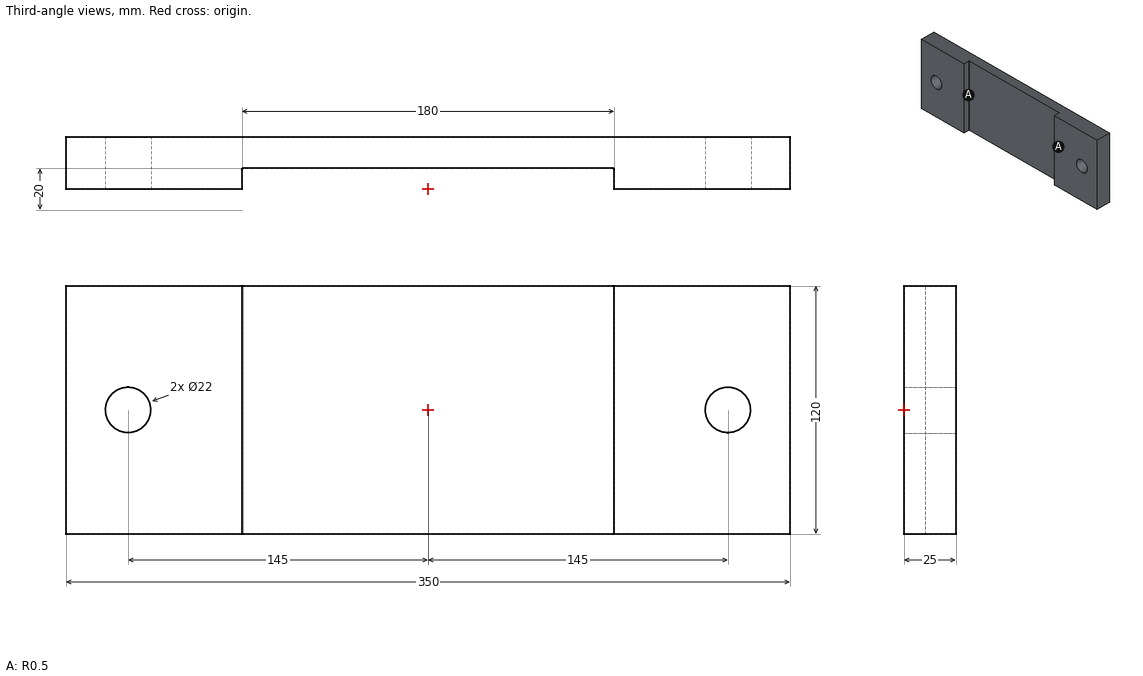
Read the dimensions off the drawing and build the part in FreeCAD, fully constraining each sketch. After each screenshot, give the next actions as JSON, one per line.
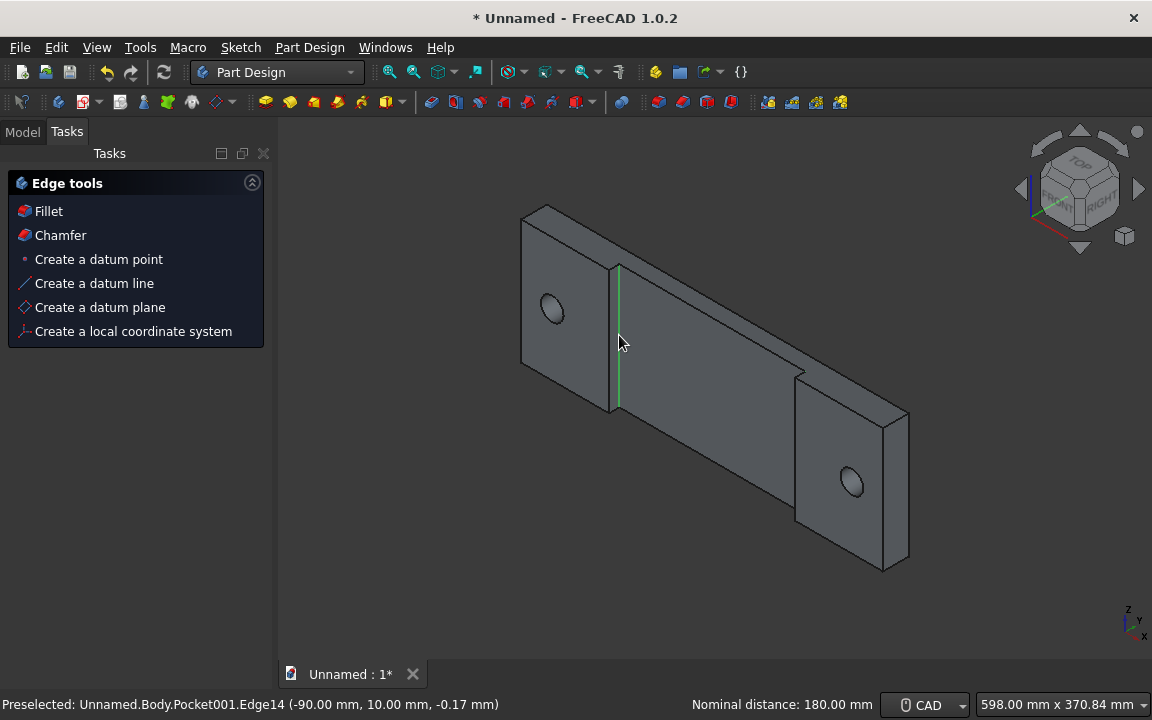
{"action": "left_click", "coordinate": [660, 102]}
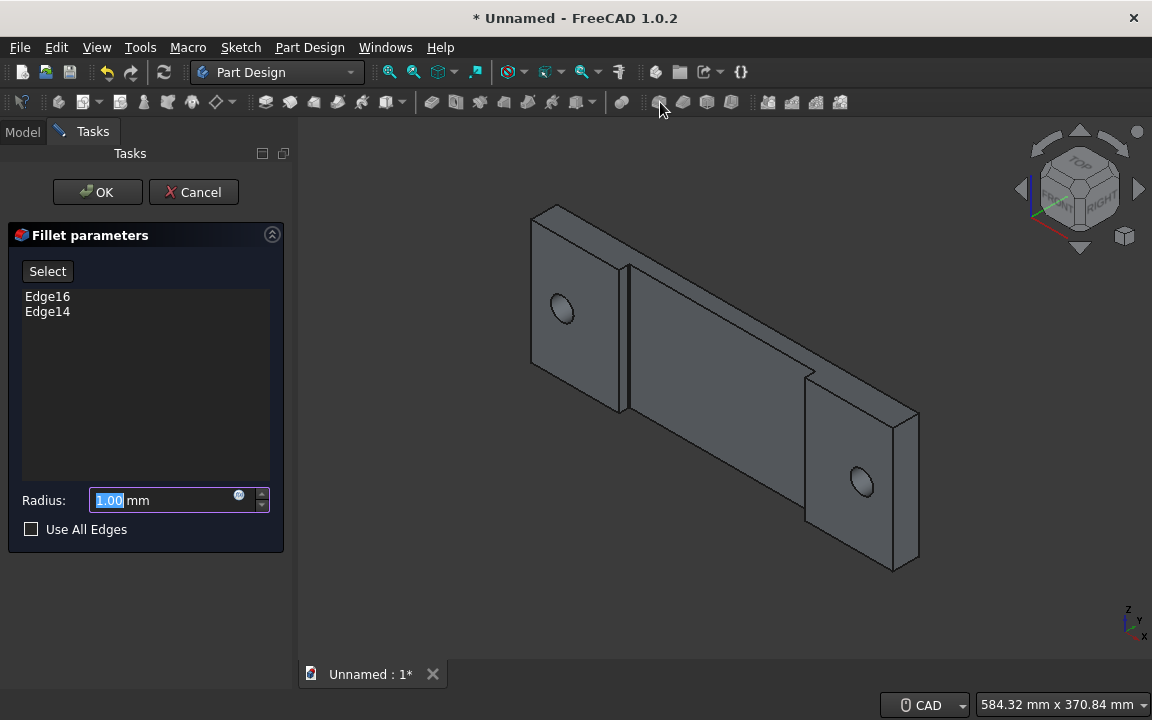
{"action": "type", "text": "0.5"}
{"action": "key", "text": "Tab"}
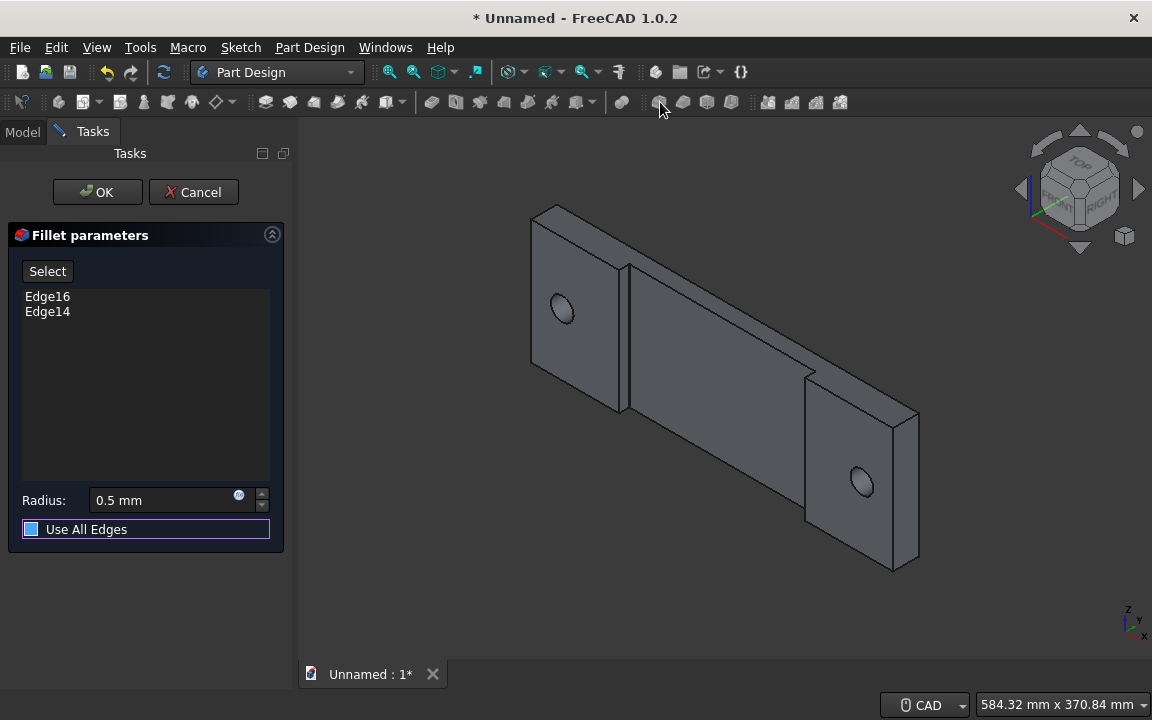
{"action": "left_click", "coordinate": [98, 192]}